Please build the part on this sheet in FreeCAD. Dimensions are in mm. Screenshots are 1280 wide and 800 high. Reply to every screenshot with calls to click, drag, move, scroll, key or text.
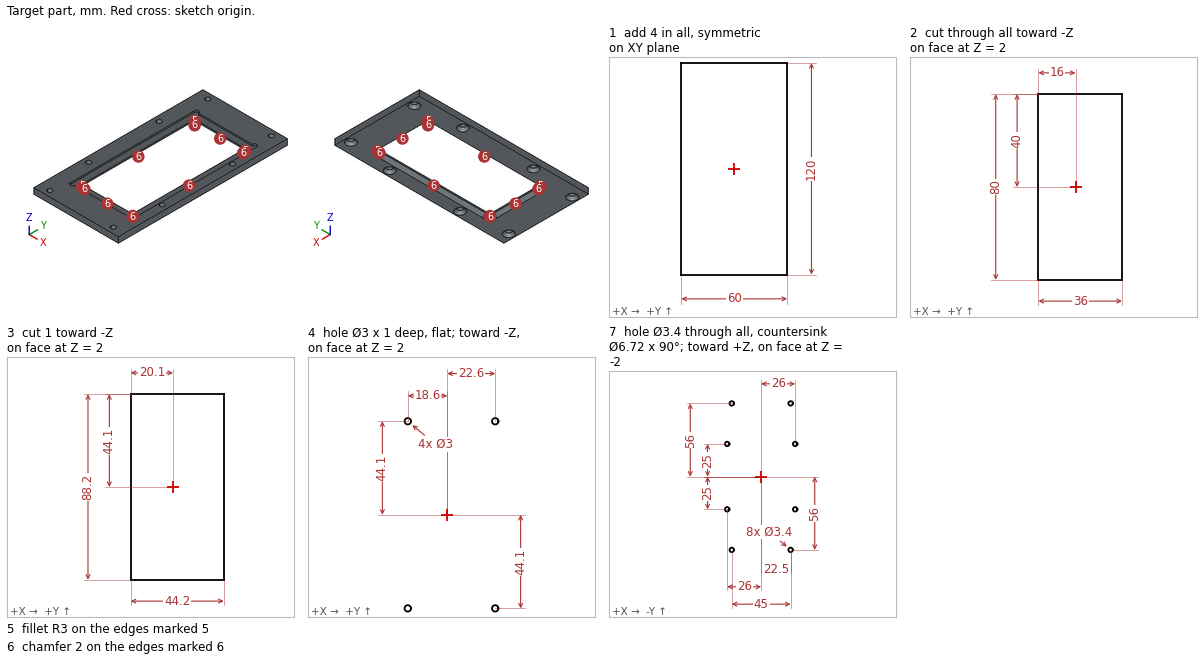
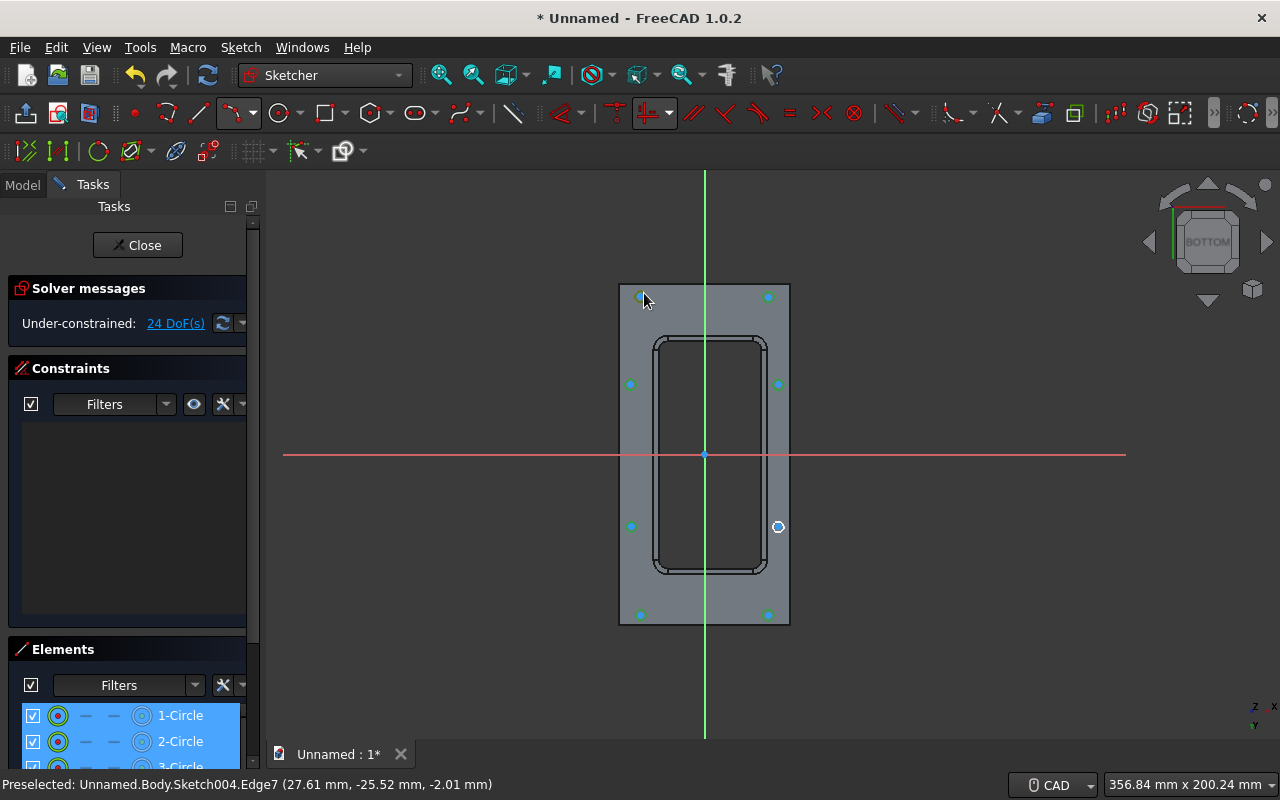
scroll(782, 523, up, 5)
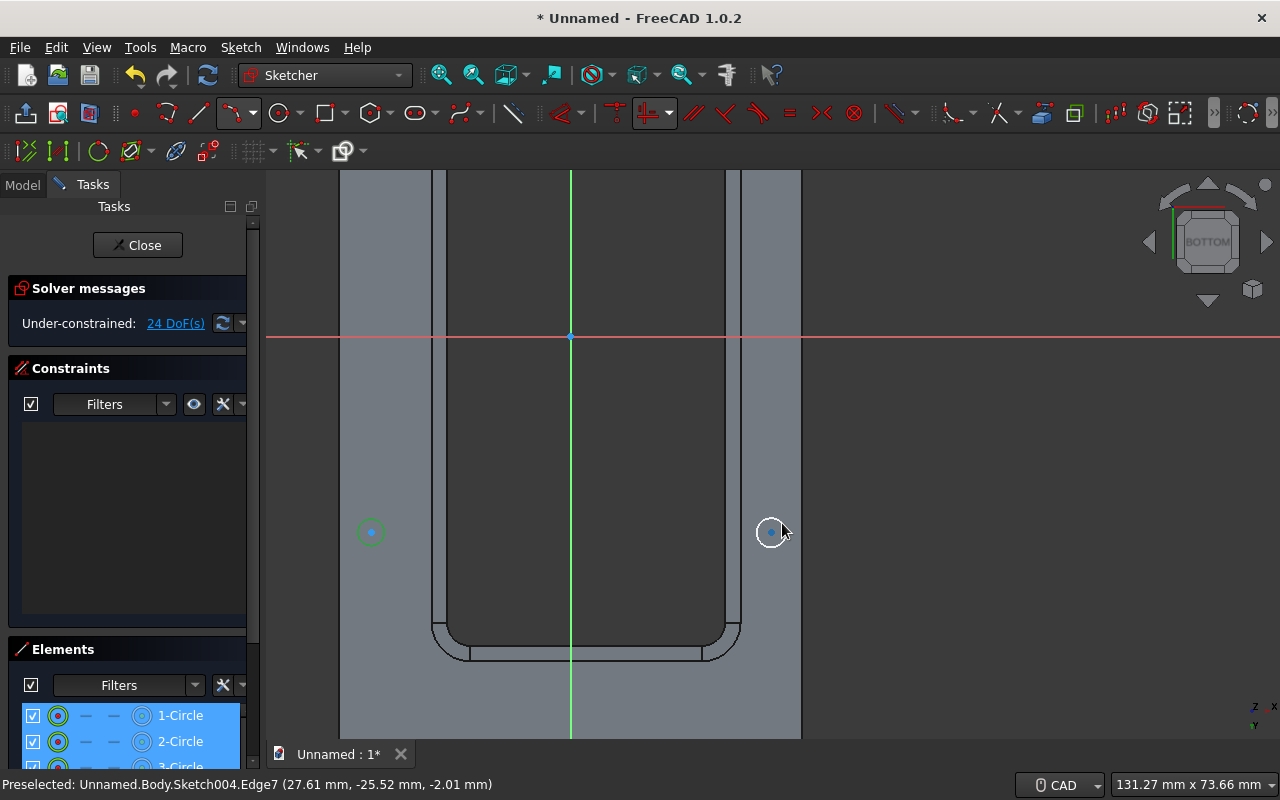
click(782, 522)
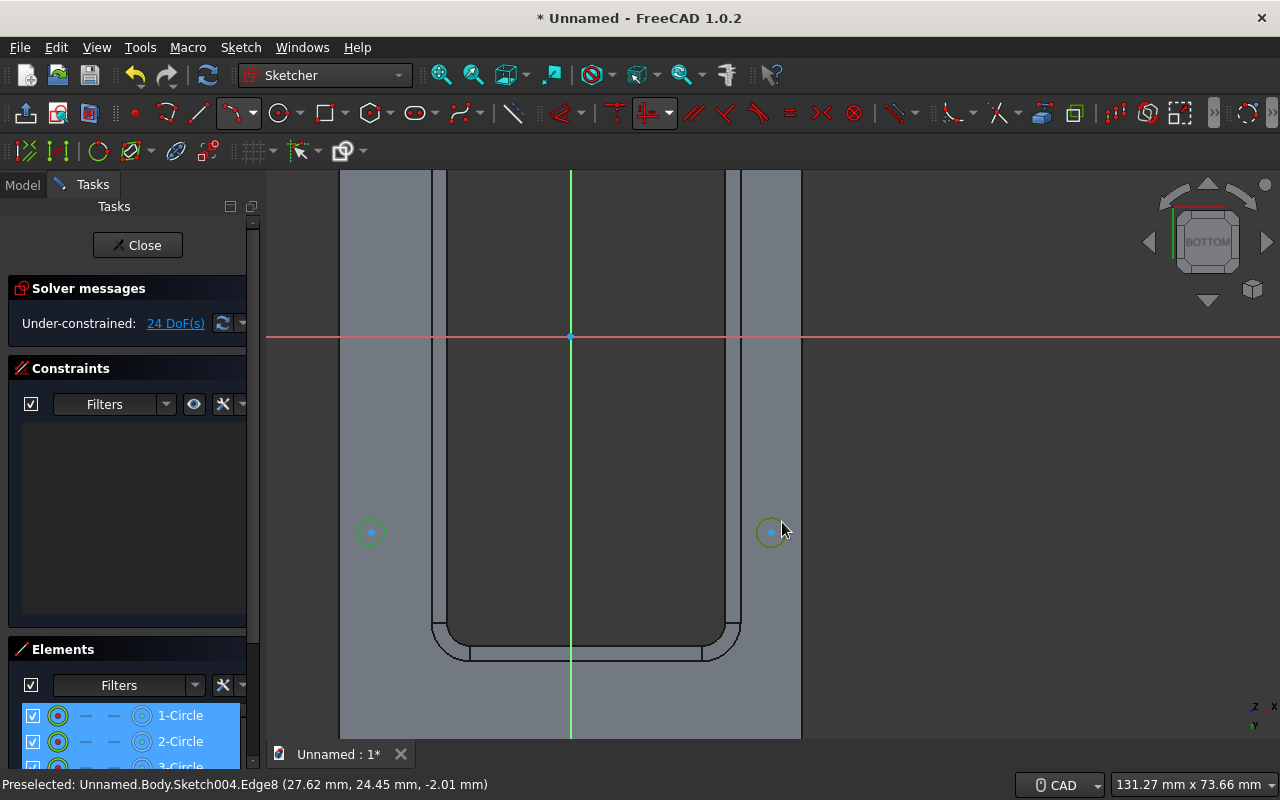
click(790, 114)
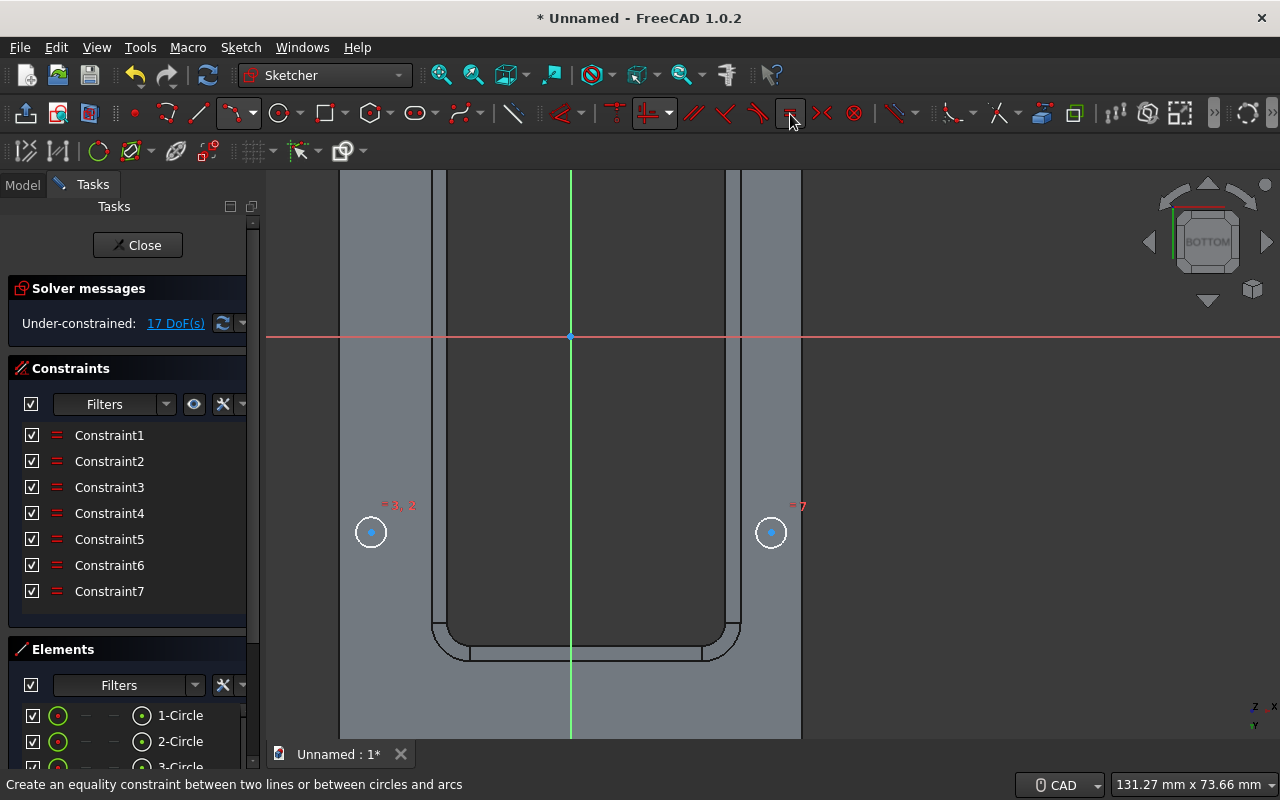
scroll(782, 523, down, 5)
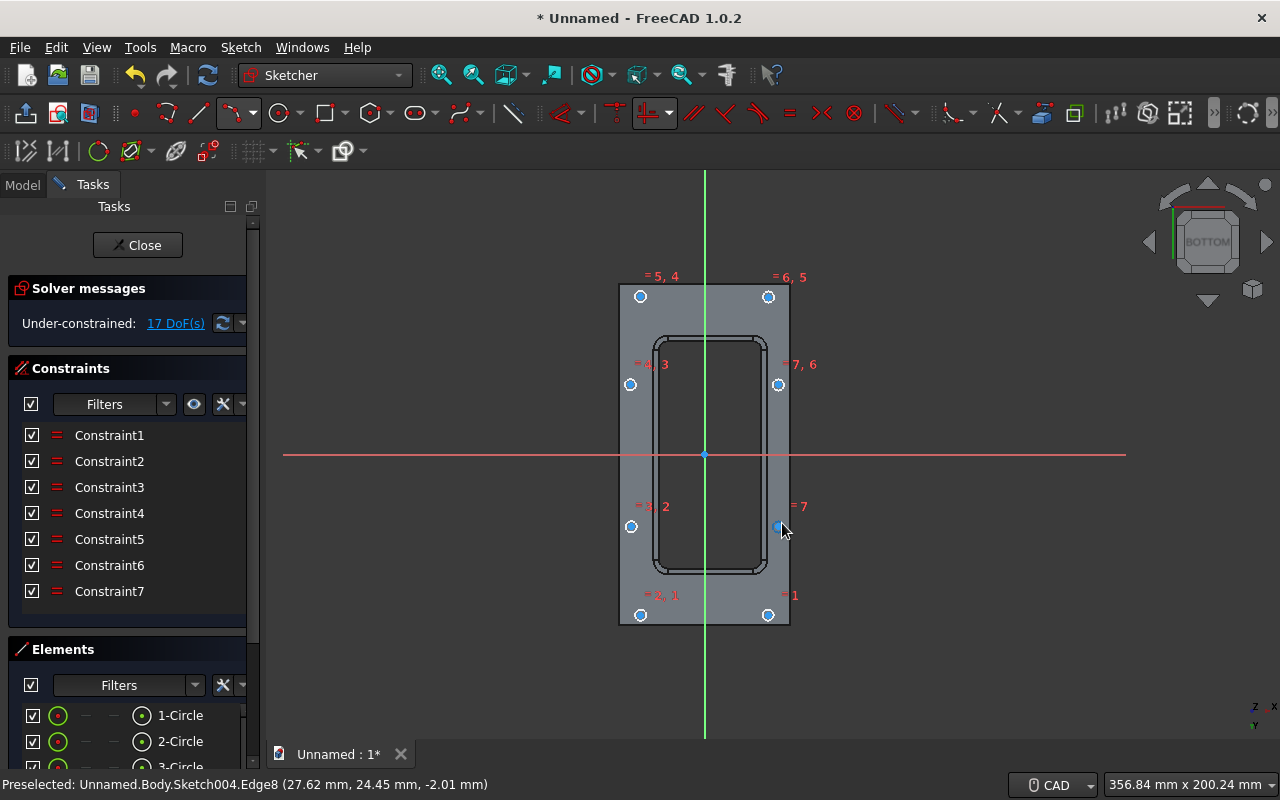
click(768, 615)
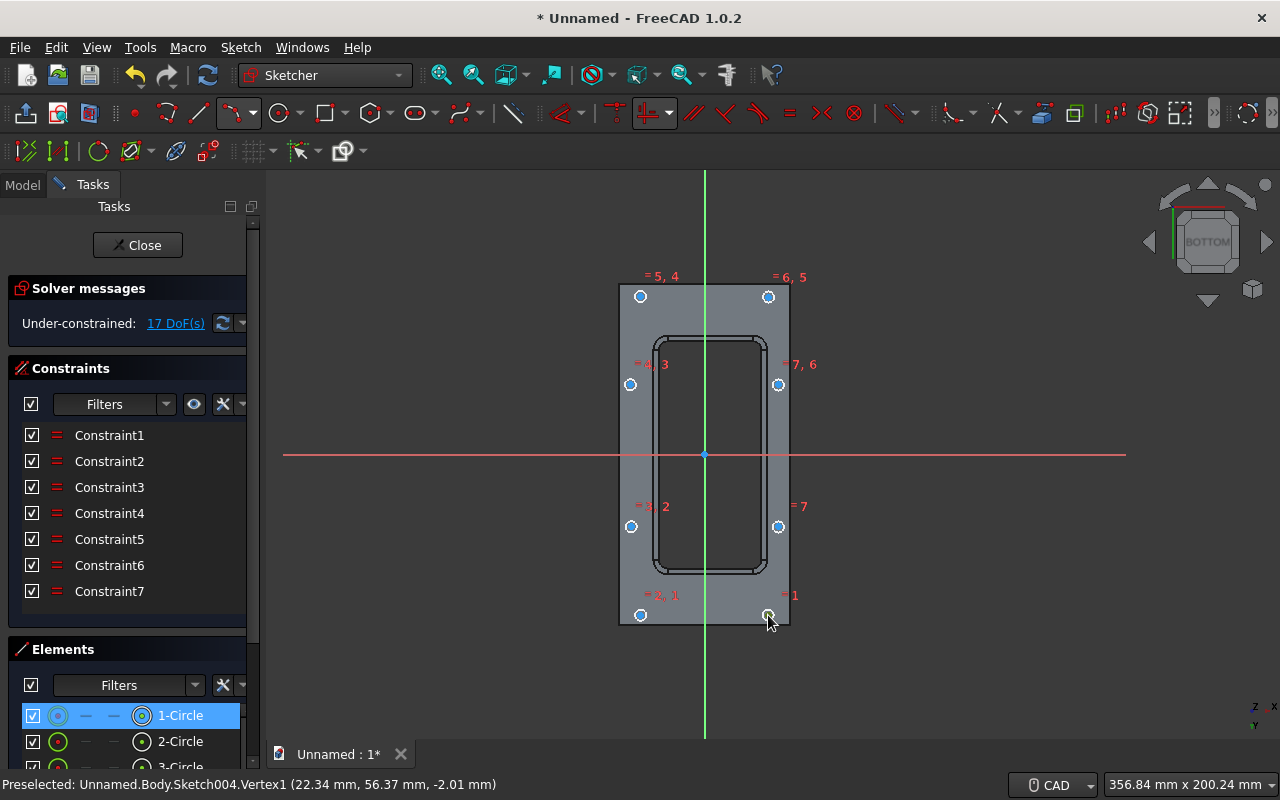
click(641, 615)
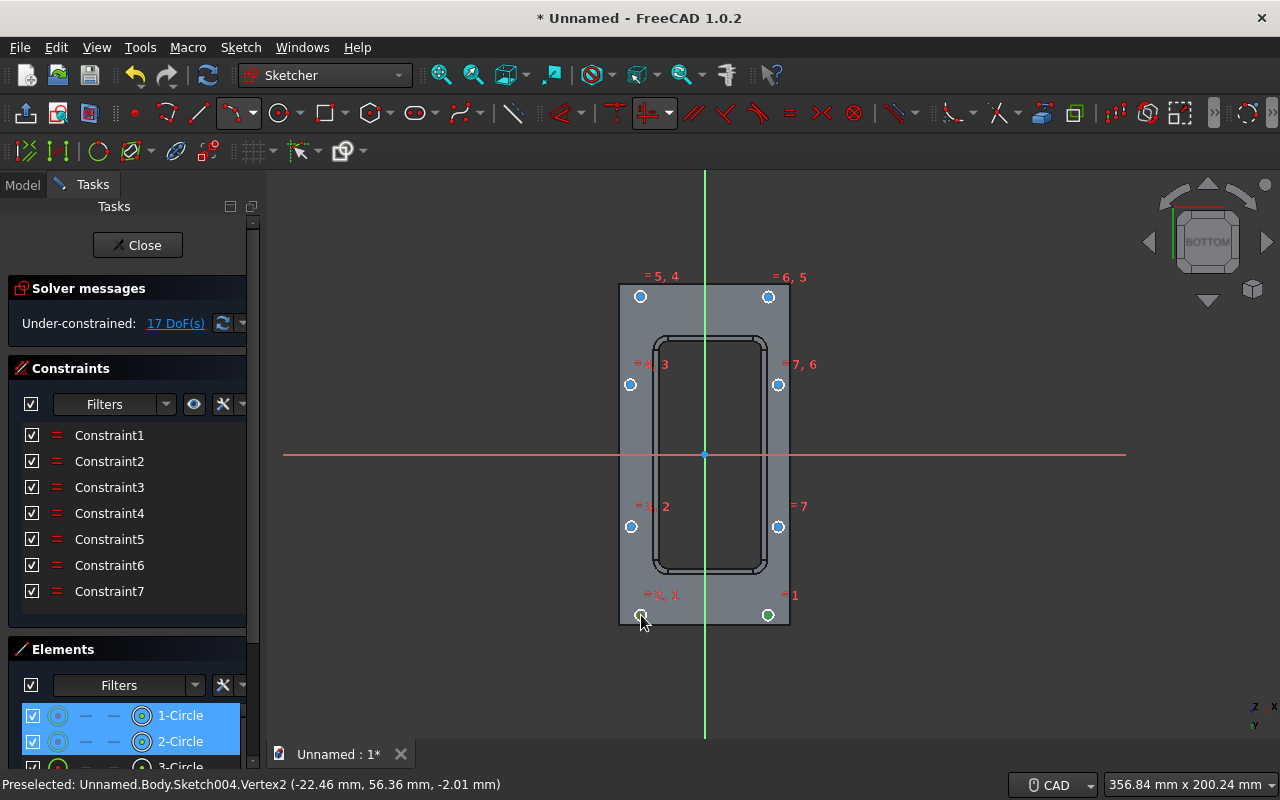
click(672, 114)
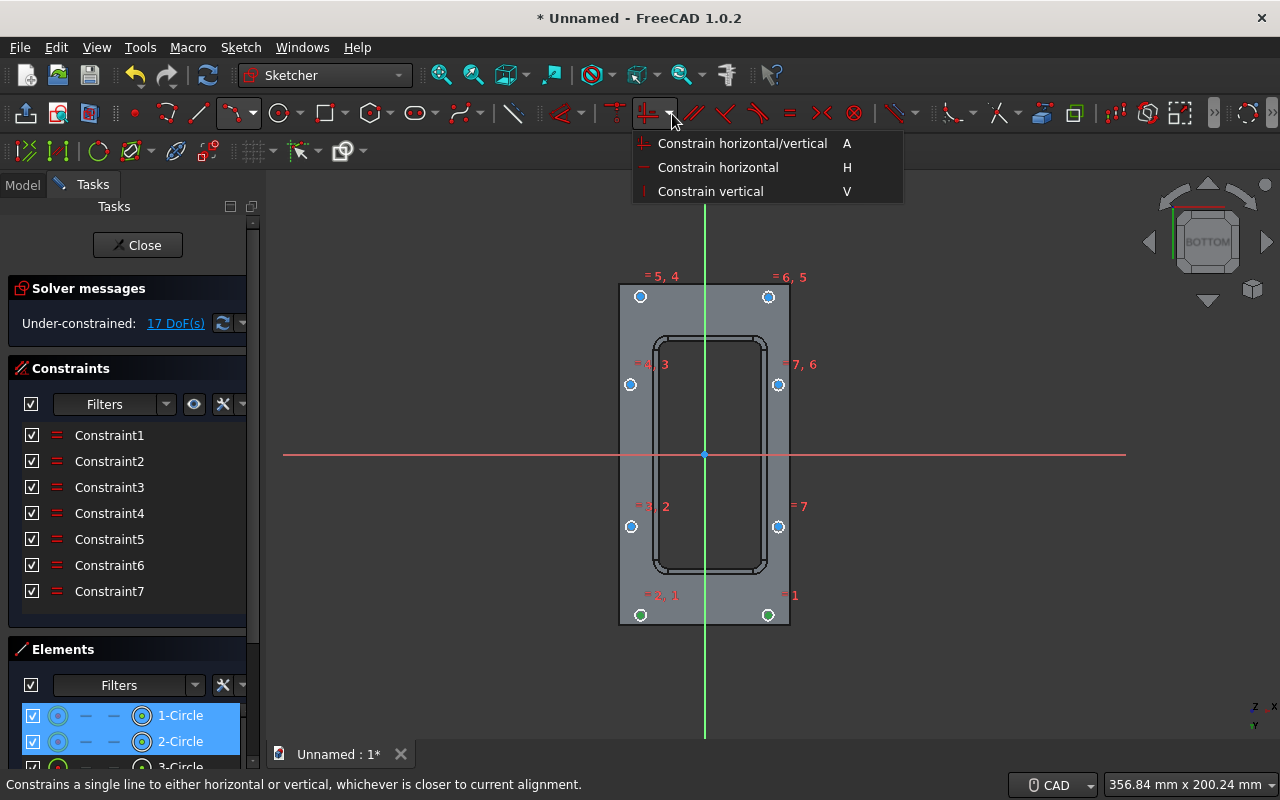
click(768, 167)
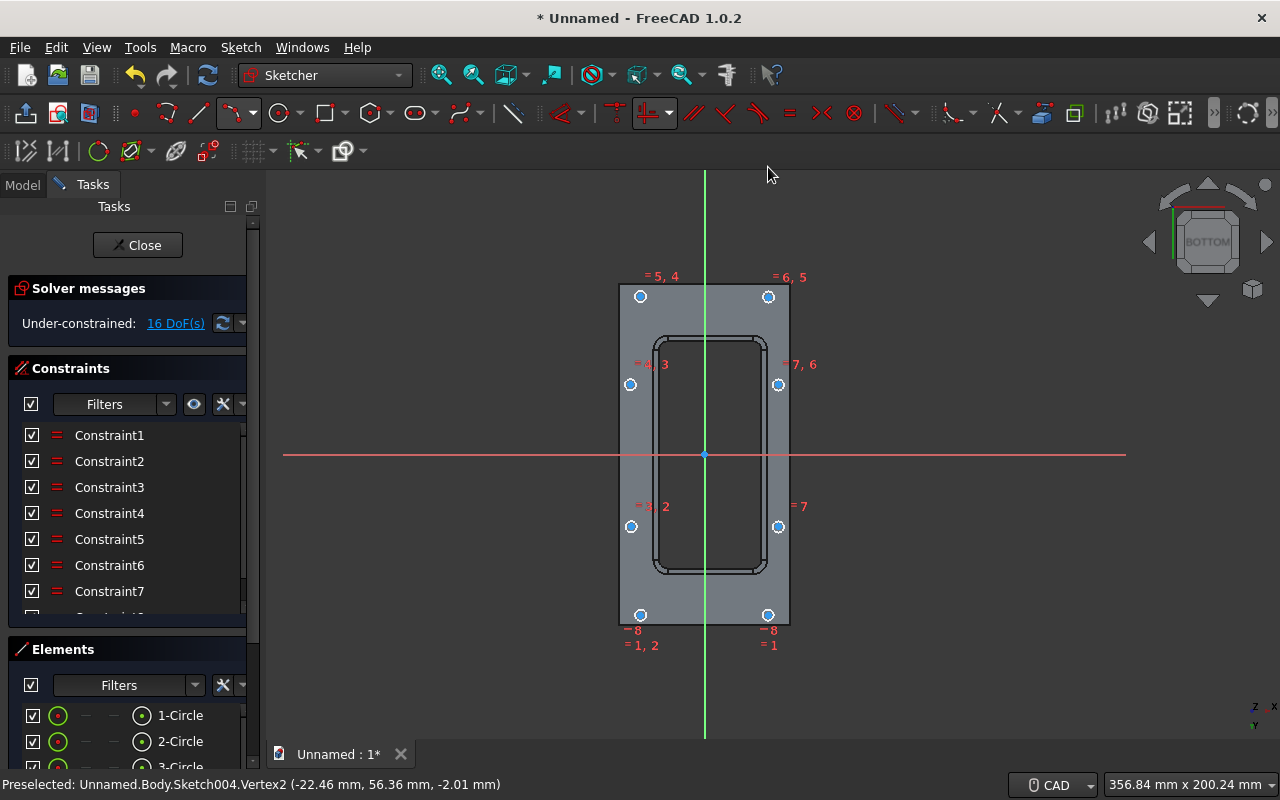
click(631, 527)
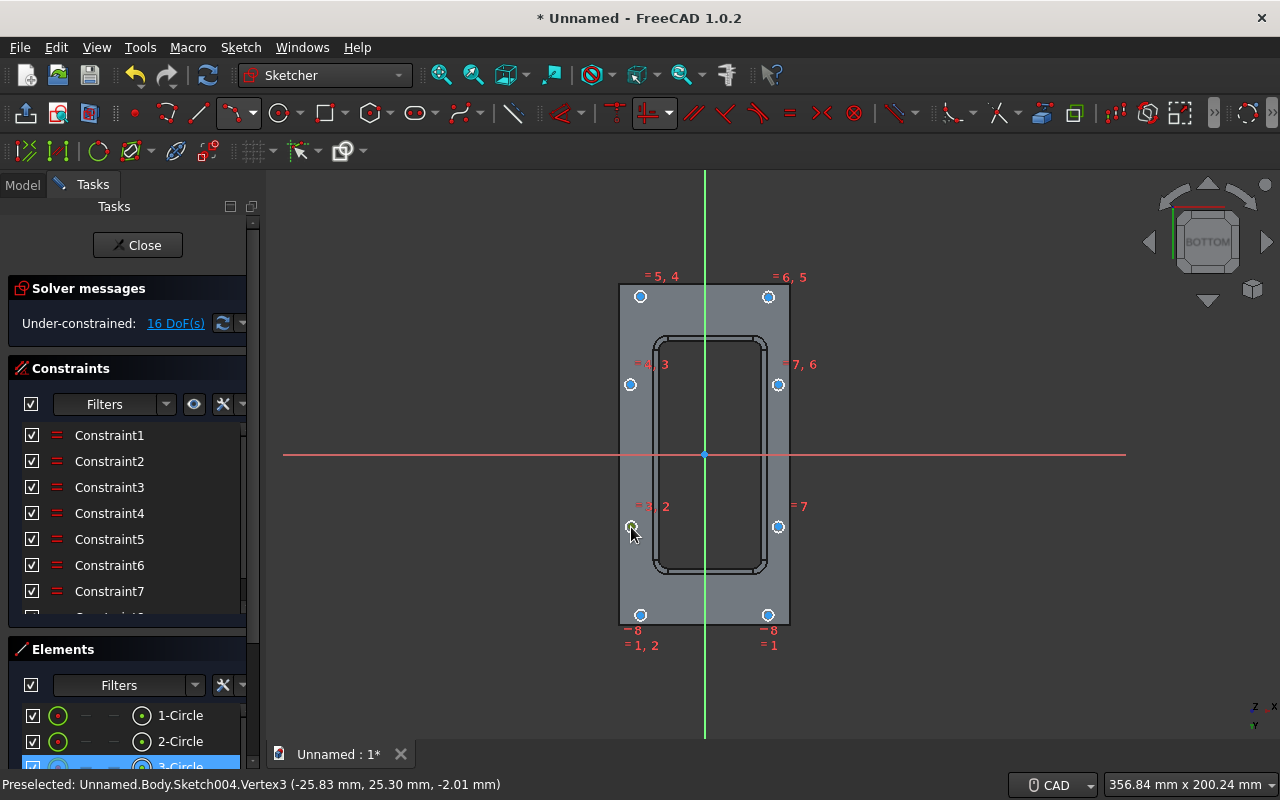
click(630, 385)